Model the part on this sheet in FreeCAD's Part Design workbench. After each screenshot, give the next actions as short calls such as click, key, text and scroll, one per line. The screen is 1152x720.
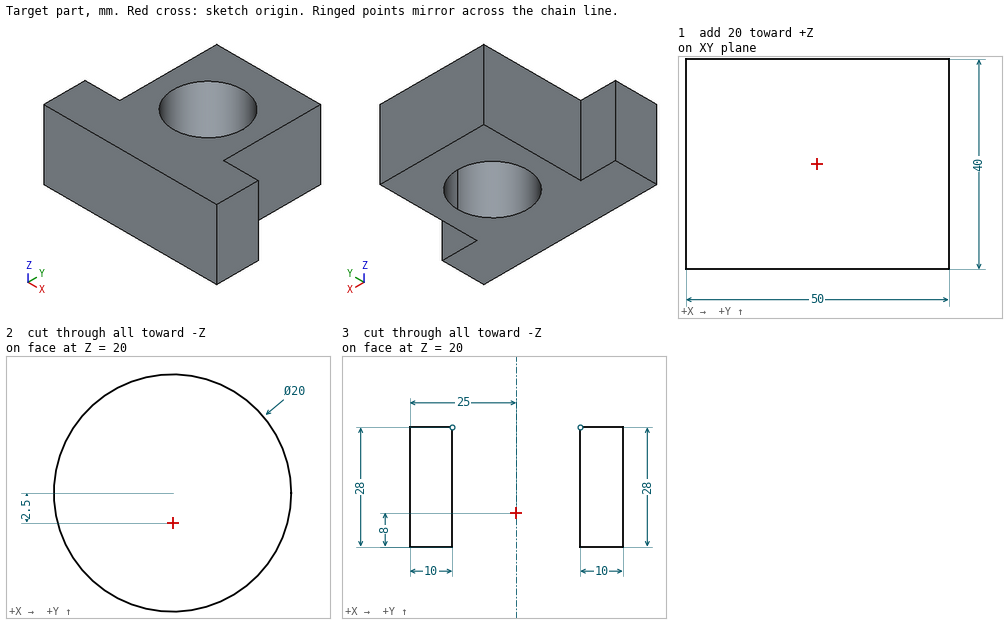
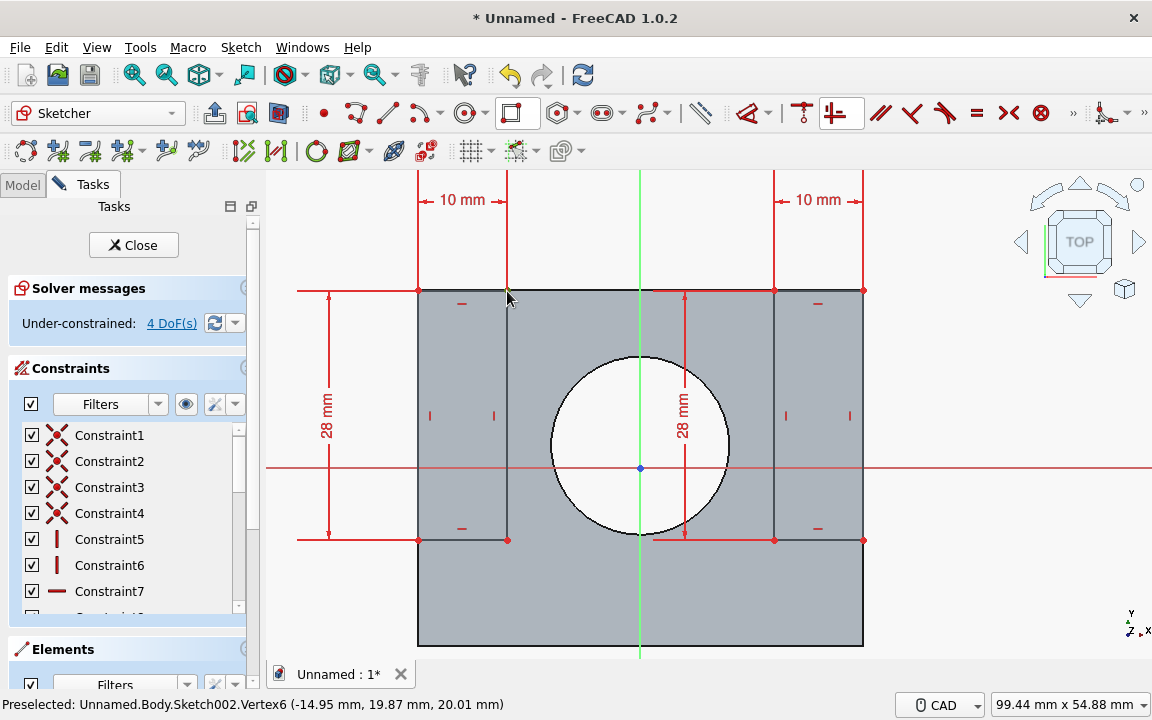
click(774, 291)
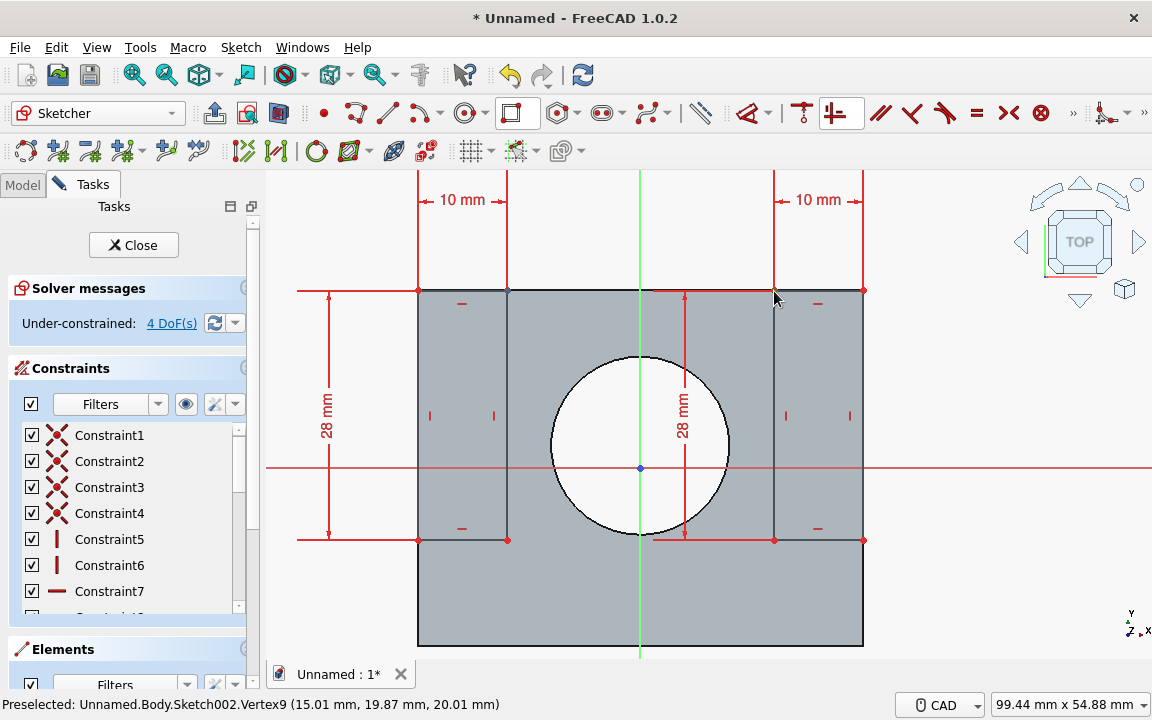
click(640, 600)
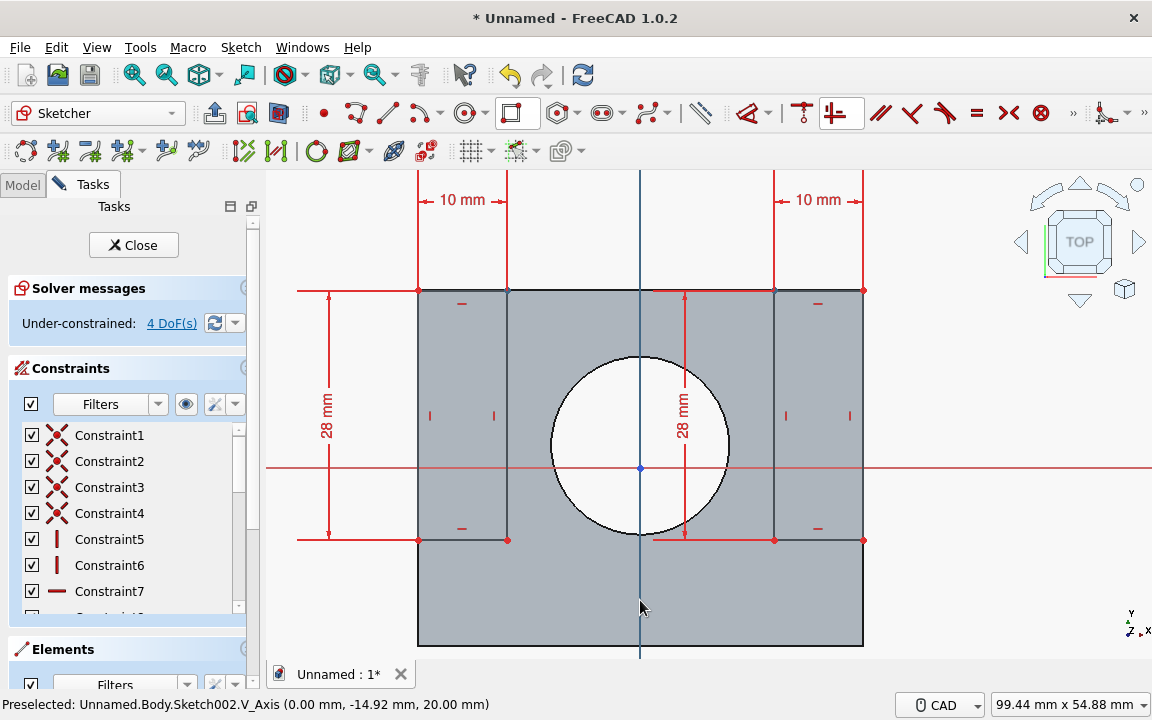
click(1010, 114)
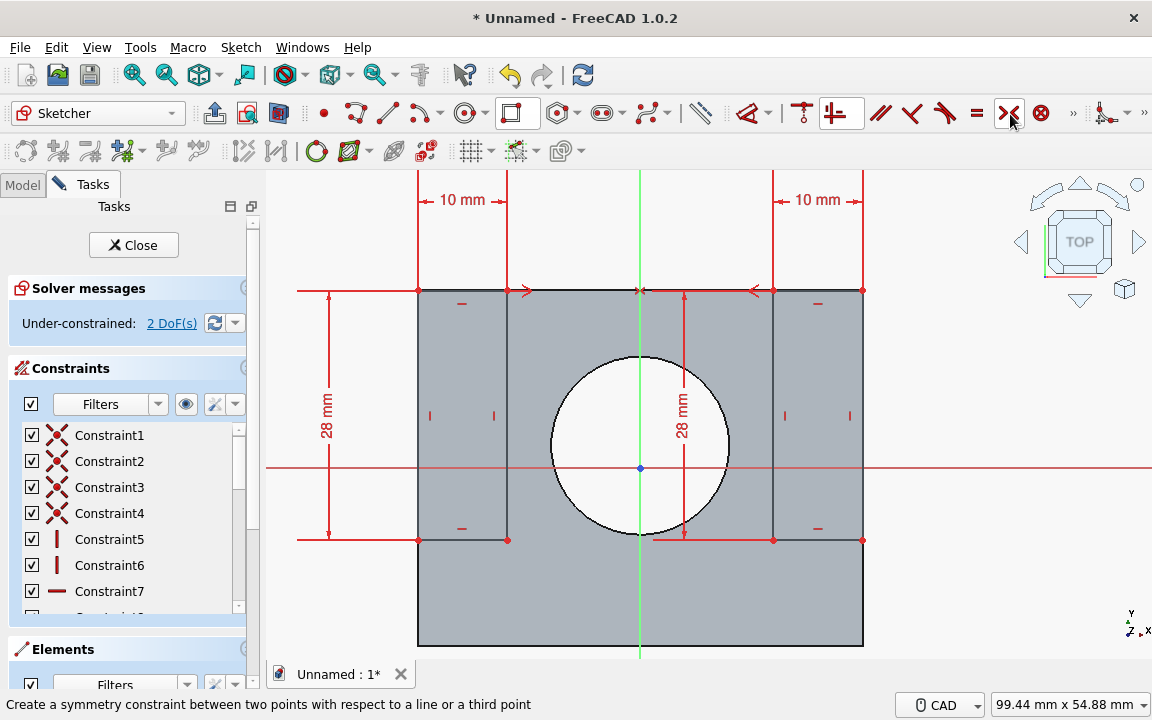
click(418, 540)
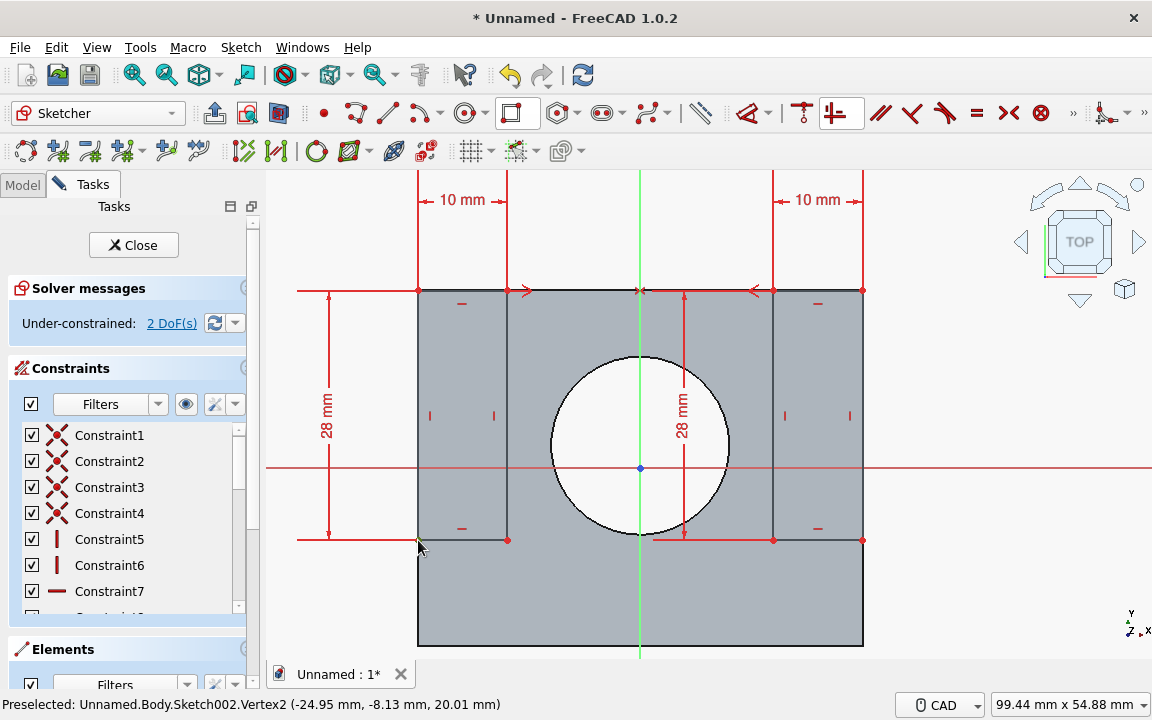
click(770, 114)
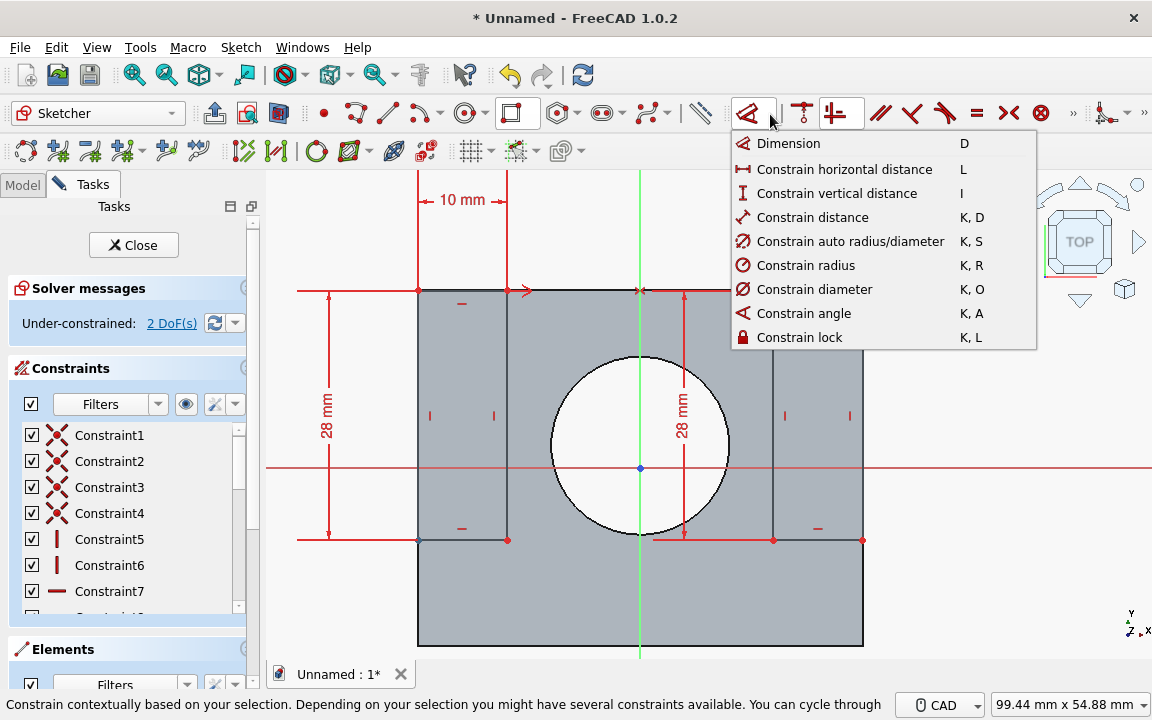
click(884, 193)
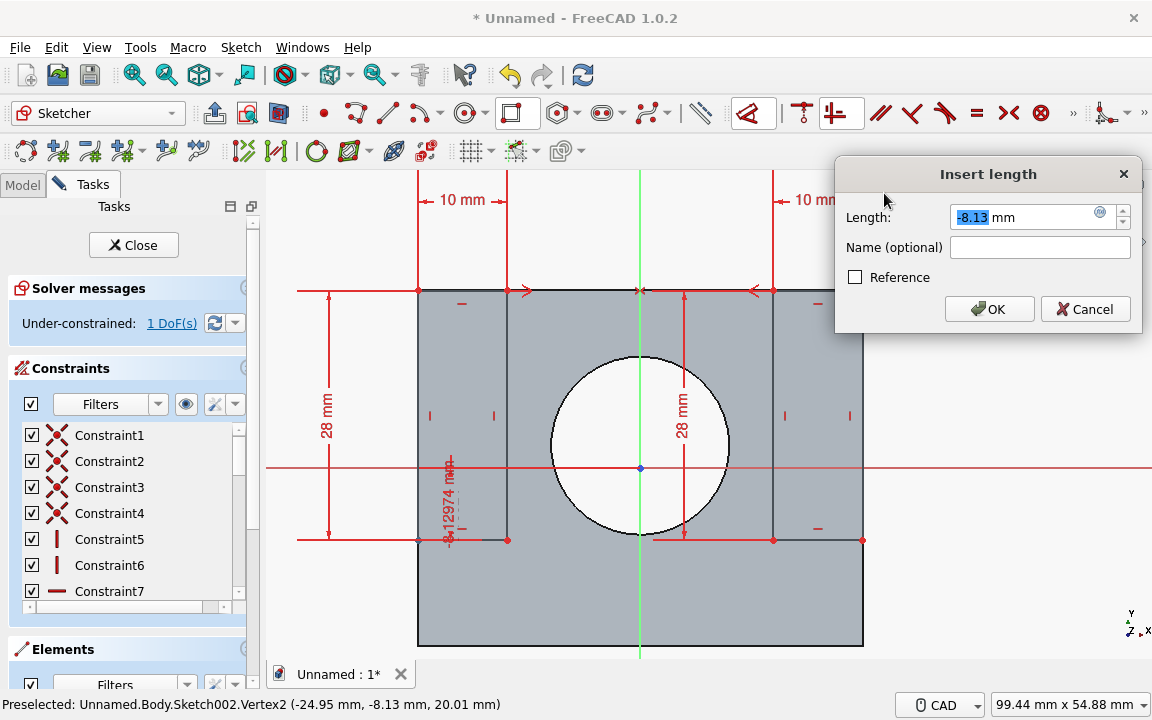
text(-8)
key(Return)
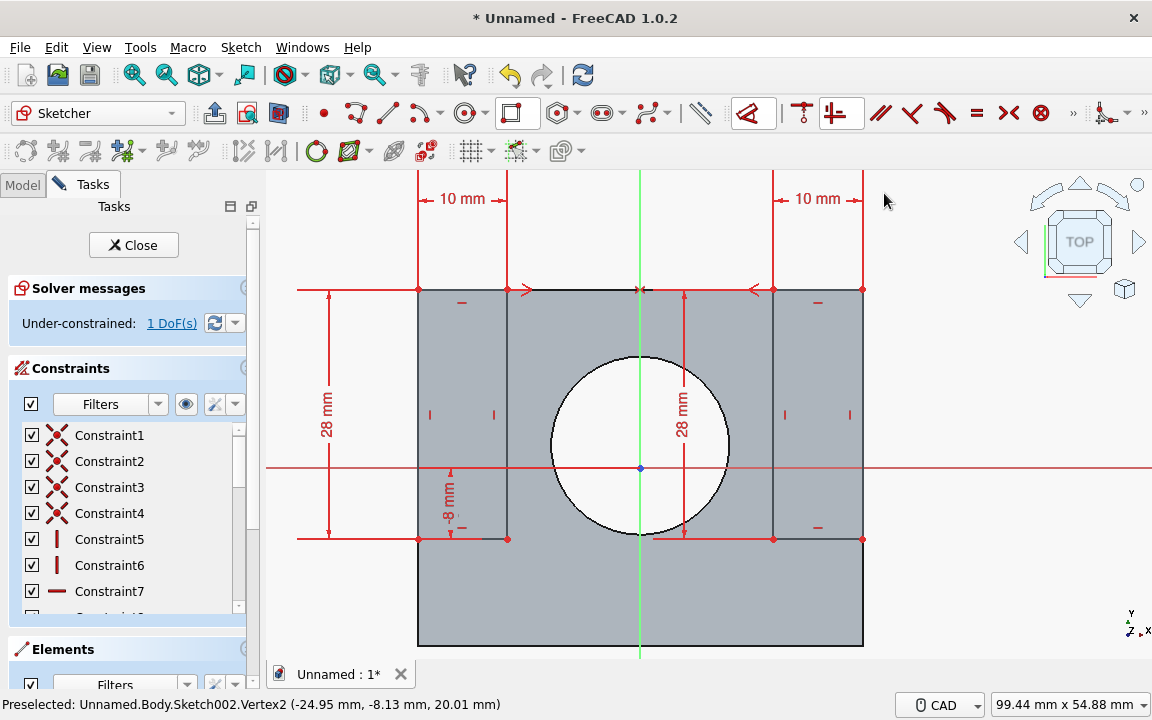
click(418, 290)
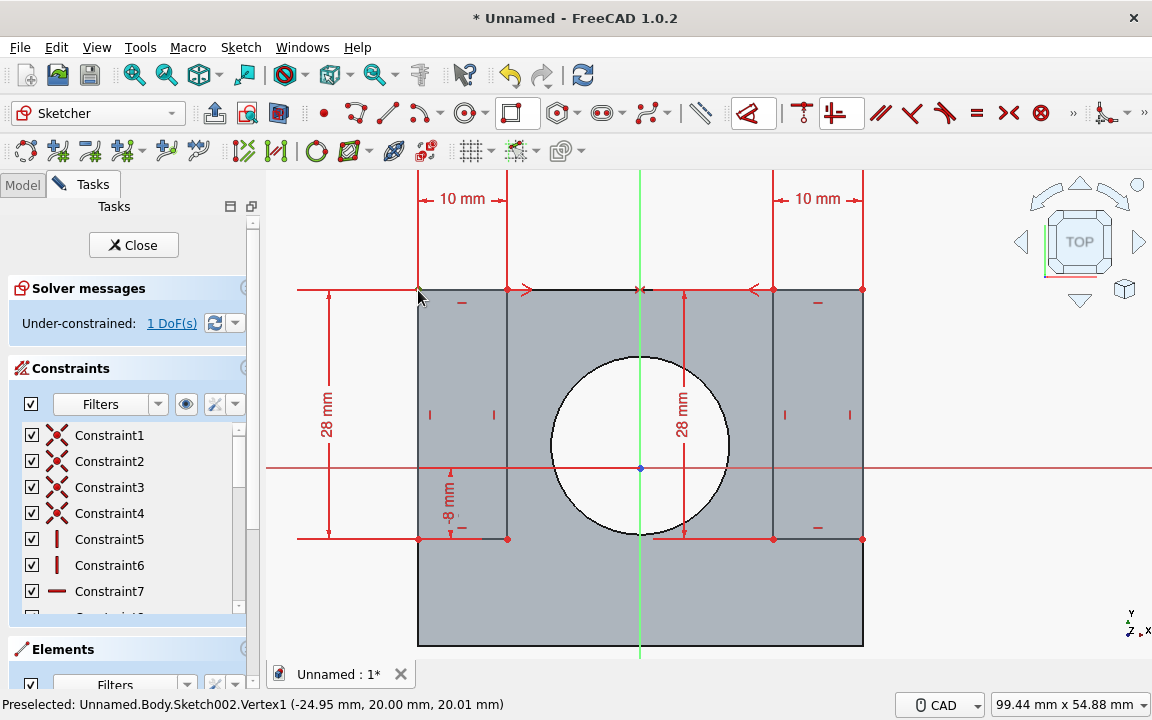
click(770, 114)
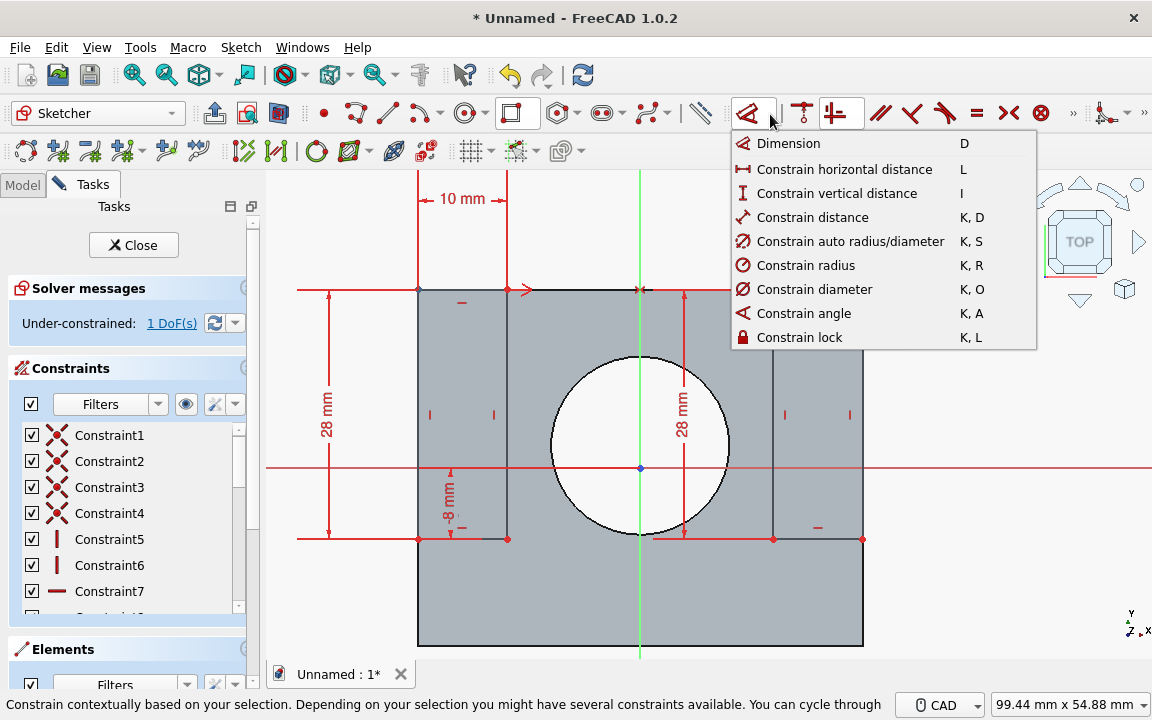
click(884, 169)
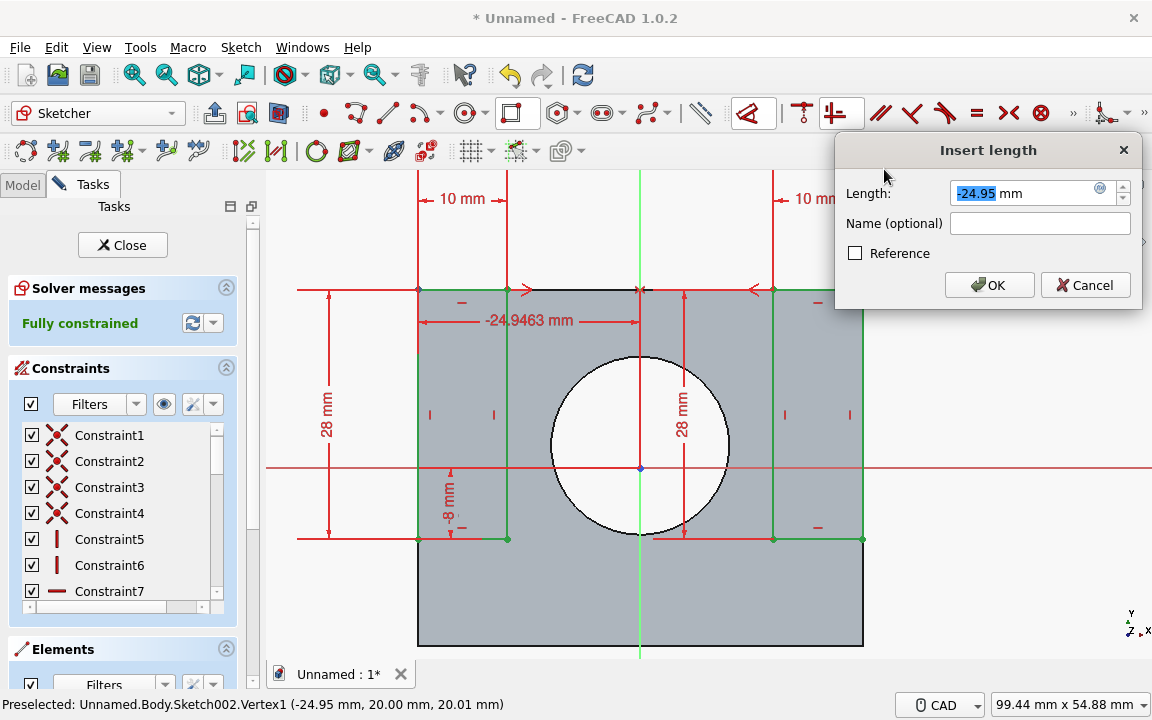
text(-25)
key(Return)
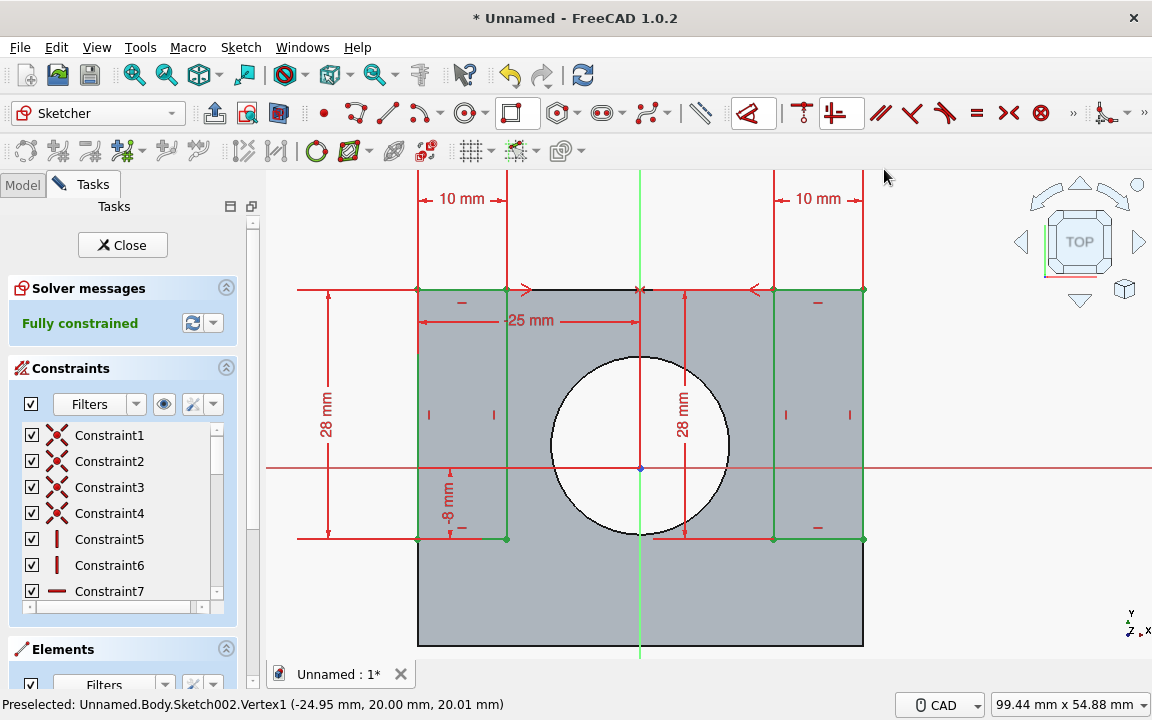
click(123, 245)